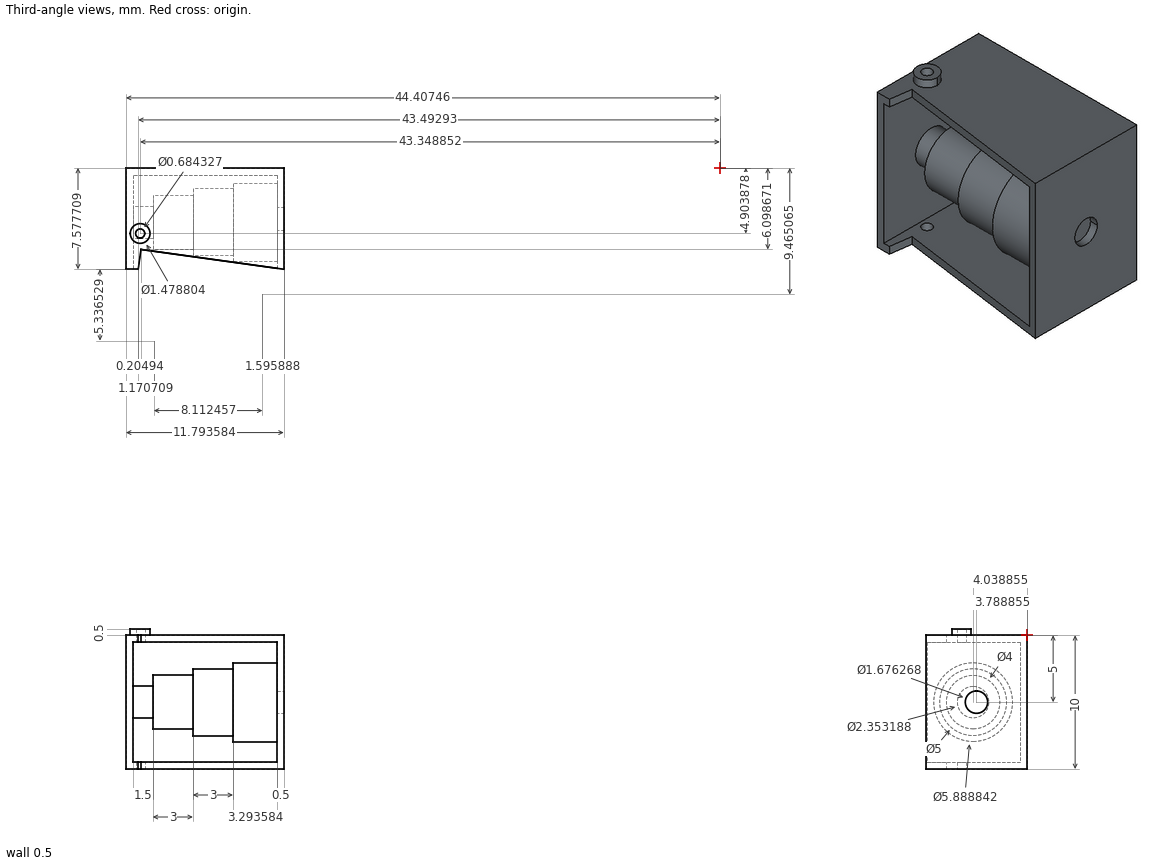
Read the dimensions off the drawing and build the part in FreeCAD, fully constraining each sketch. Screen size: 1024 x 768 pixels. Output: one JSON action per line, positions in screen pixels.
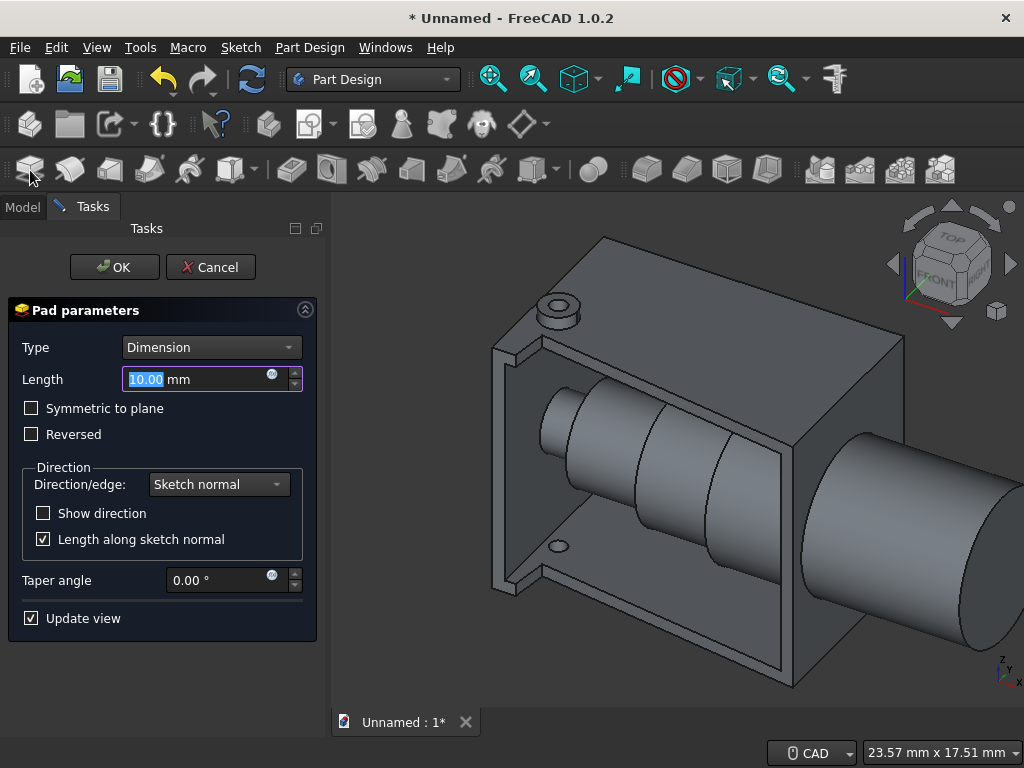
{"action": "type", "text": "3.293584"}
{"action": "key", "text": "Tab"}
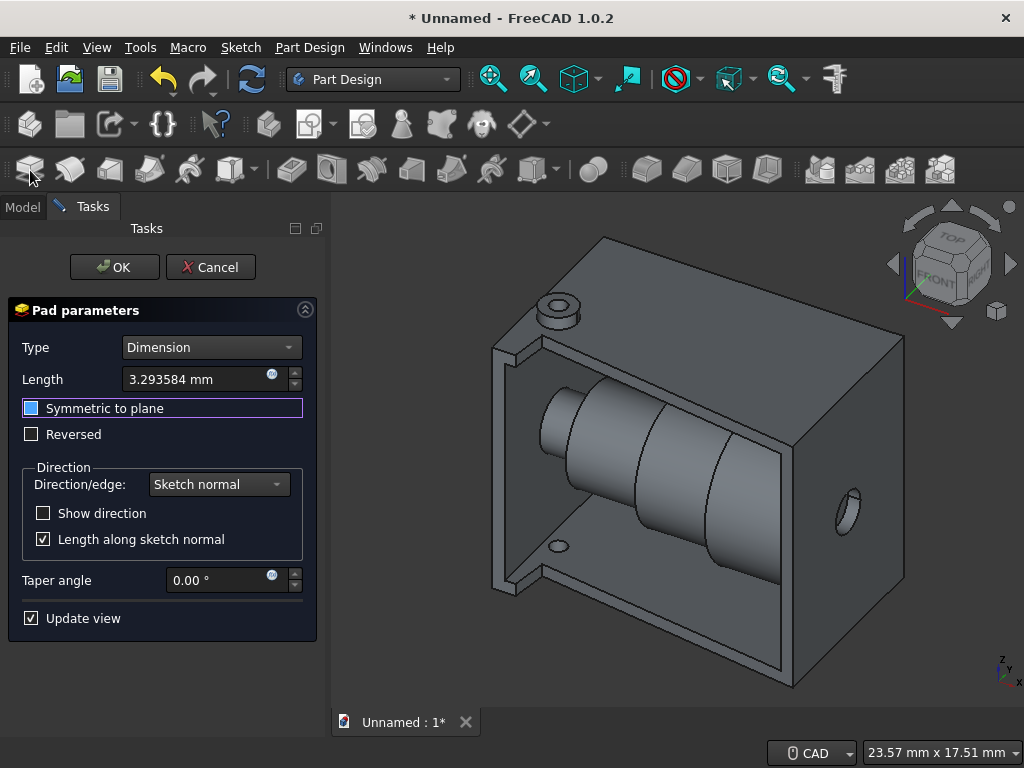
{"action": "left_click", "coordinate": [115, 267]}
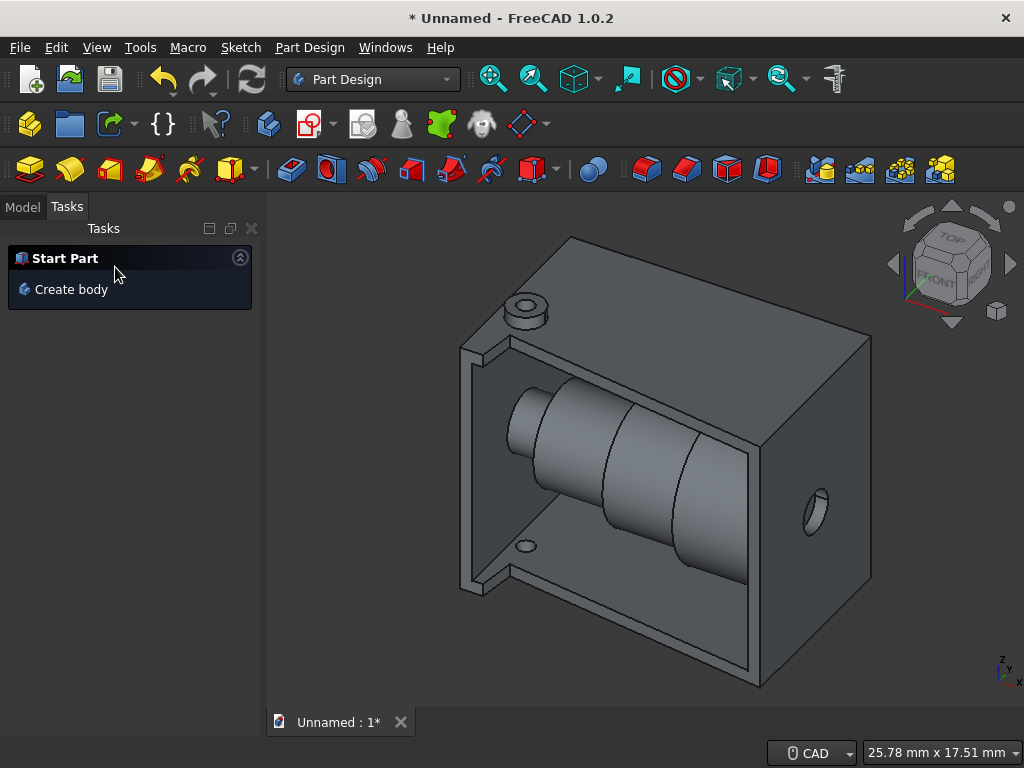
{"action": "key", "text": "0"}